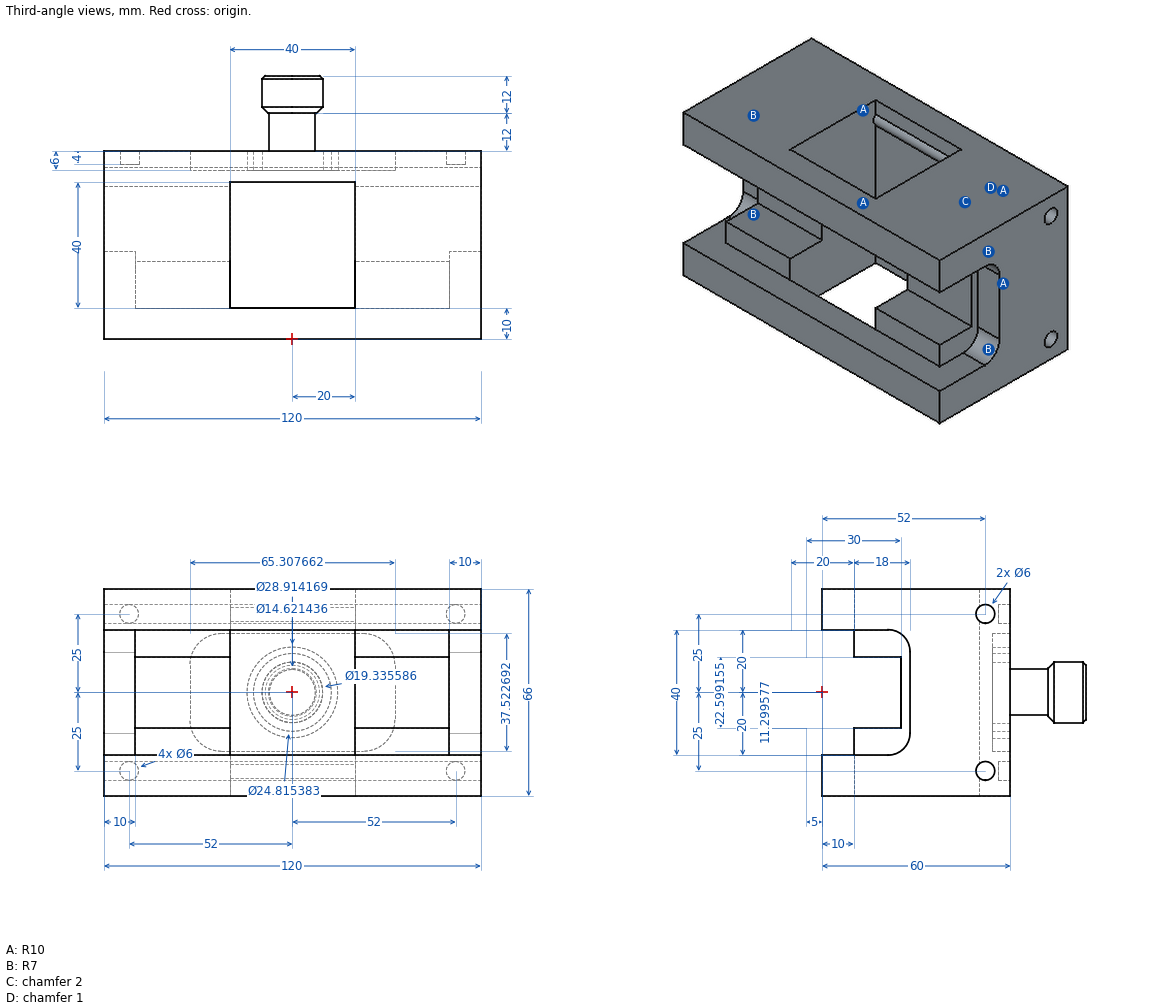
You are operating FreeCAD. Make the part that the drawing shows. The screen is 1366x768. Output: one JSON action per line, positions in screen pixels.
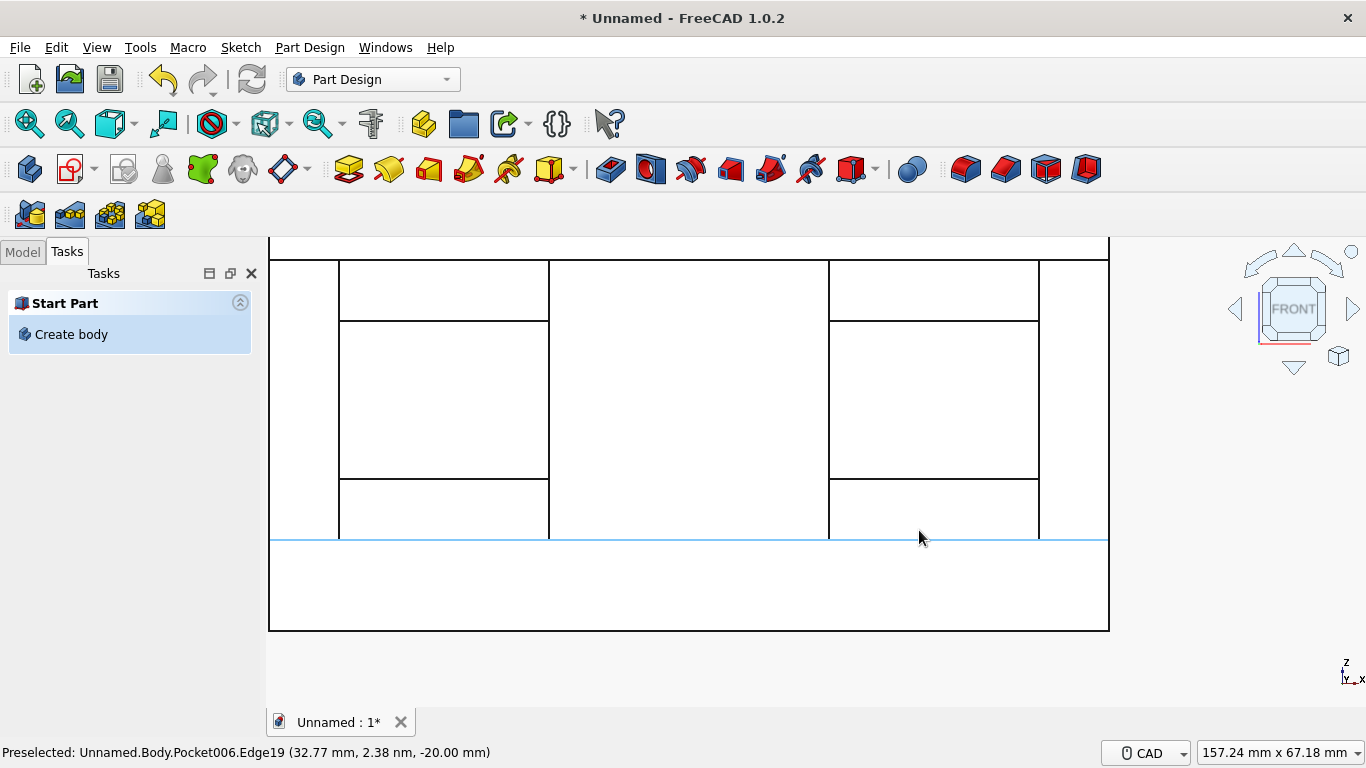
{"action": "left_click", "coordinate": [30, 124]}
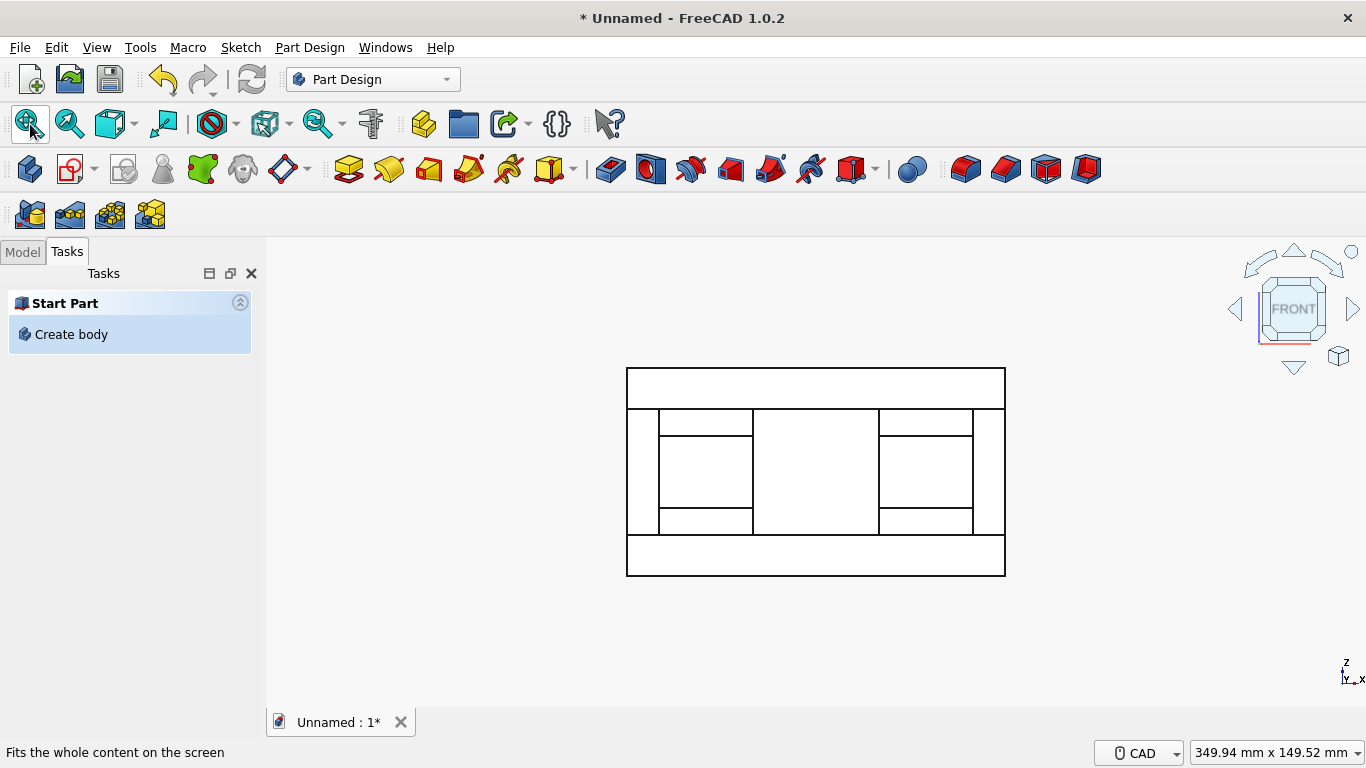
{"action": "key", "text": "3"}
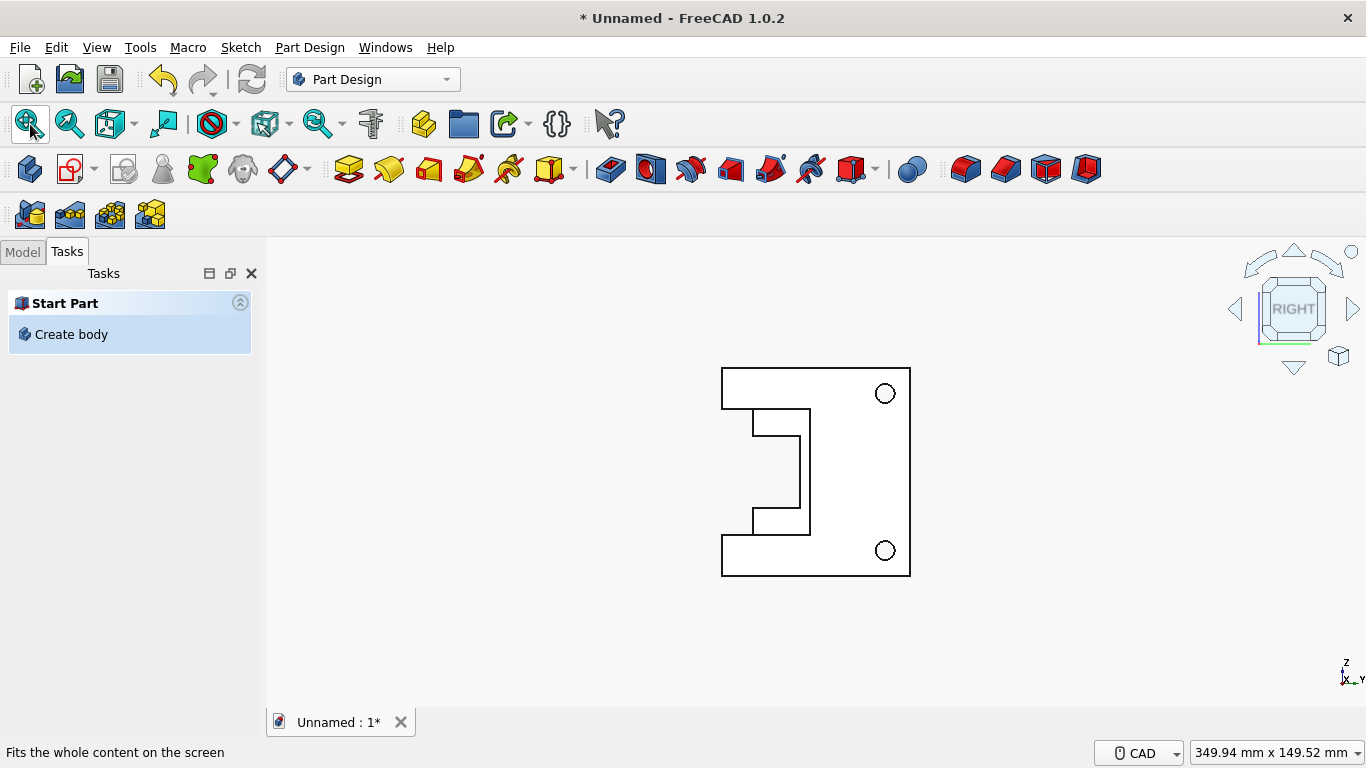
{"action": "left_click", "coordinate": [30, 124]}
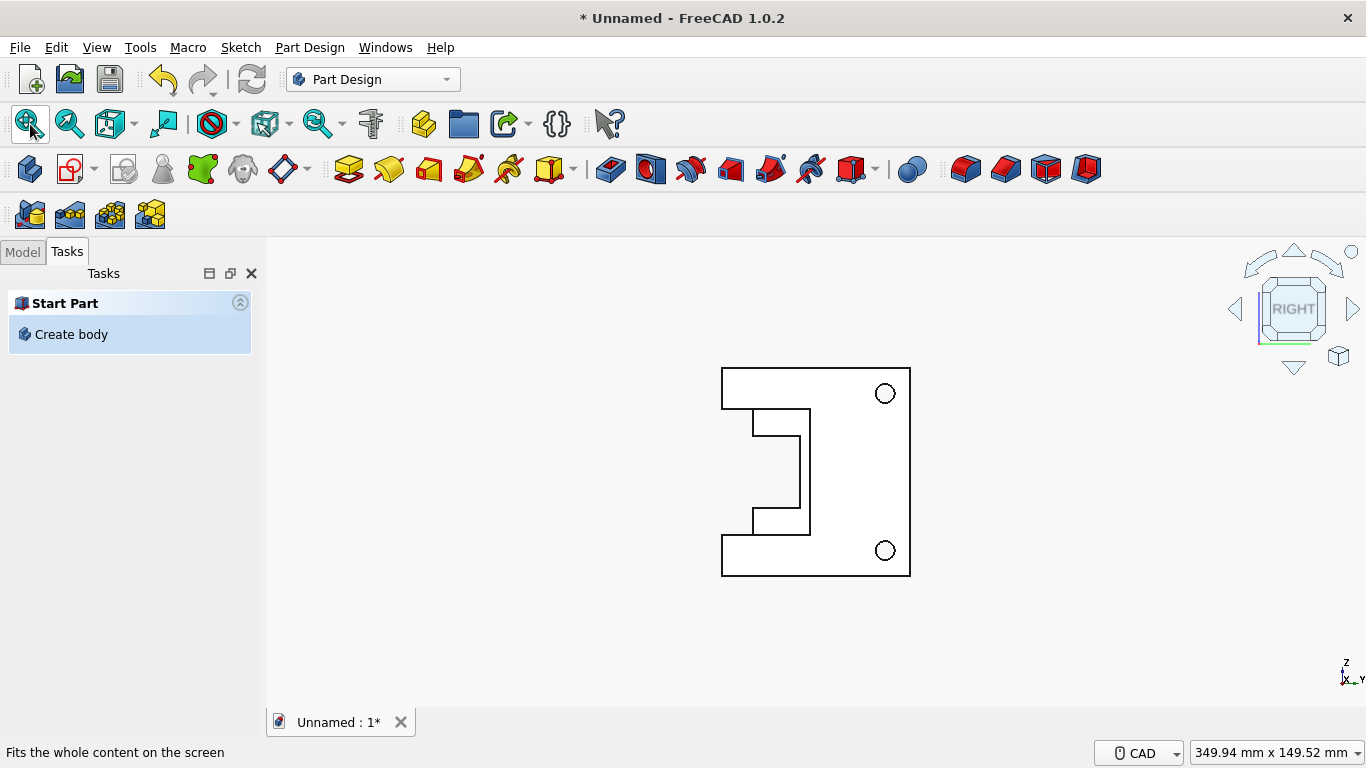
{"action": "scroll", "coordinate": [901, 530], "scroll_direction": "up", "scroll_amount": 4}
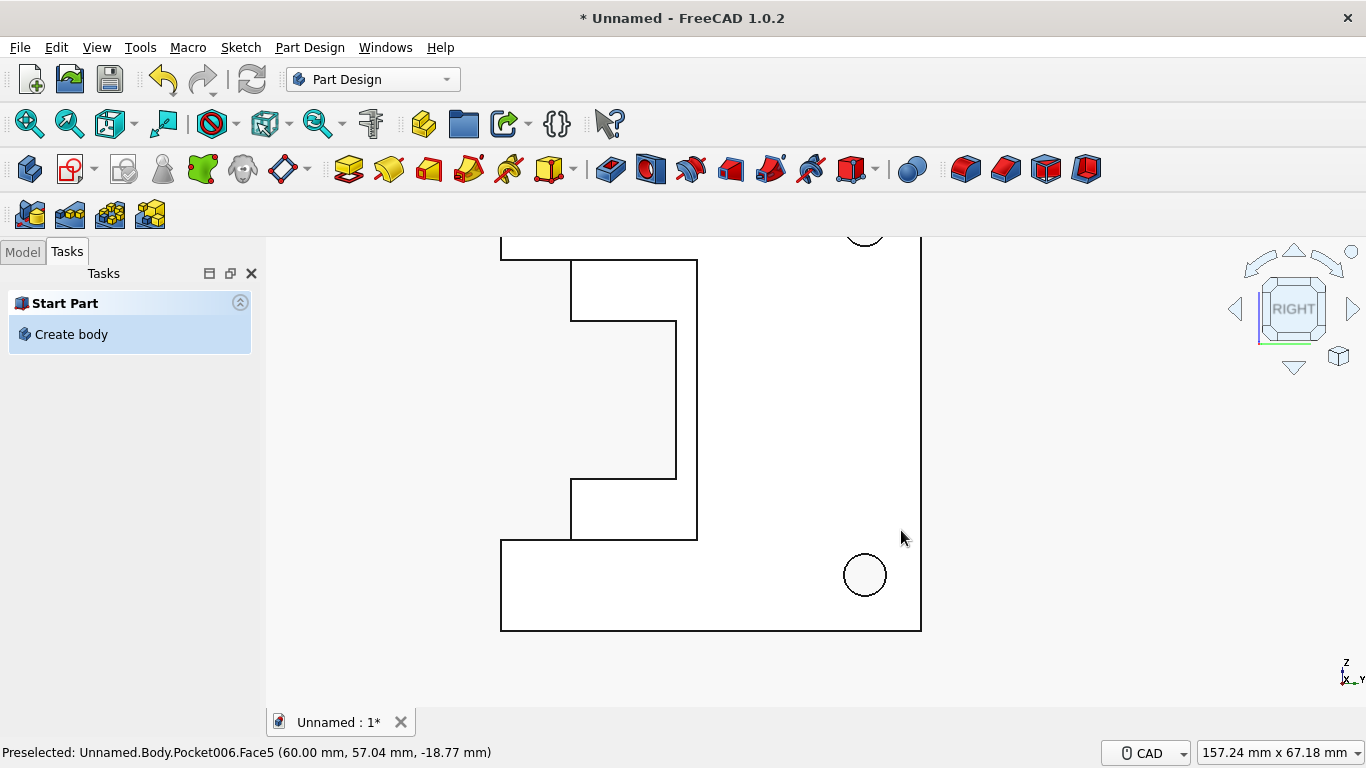
{"action": "left_click", "coordinate": [30, 124]}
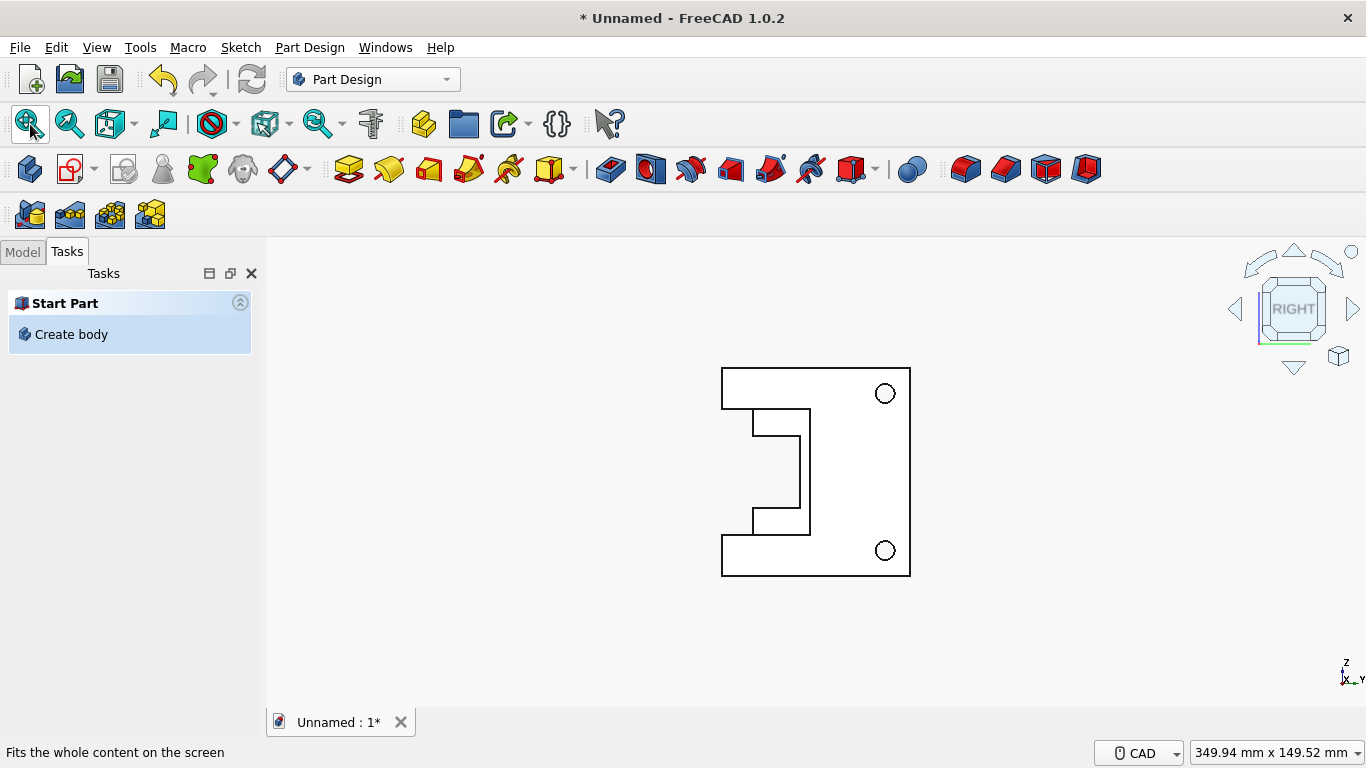
{"action": "key", "text": "5"}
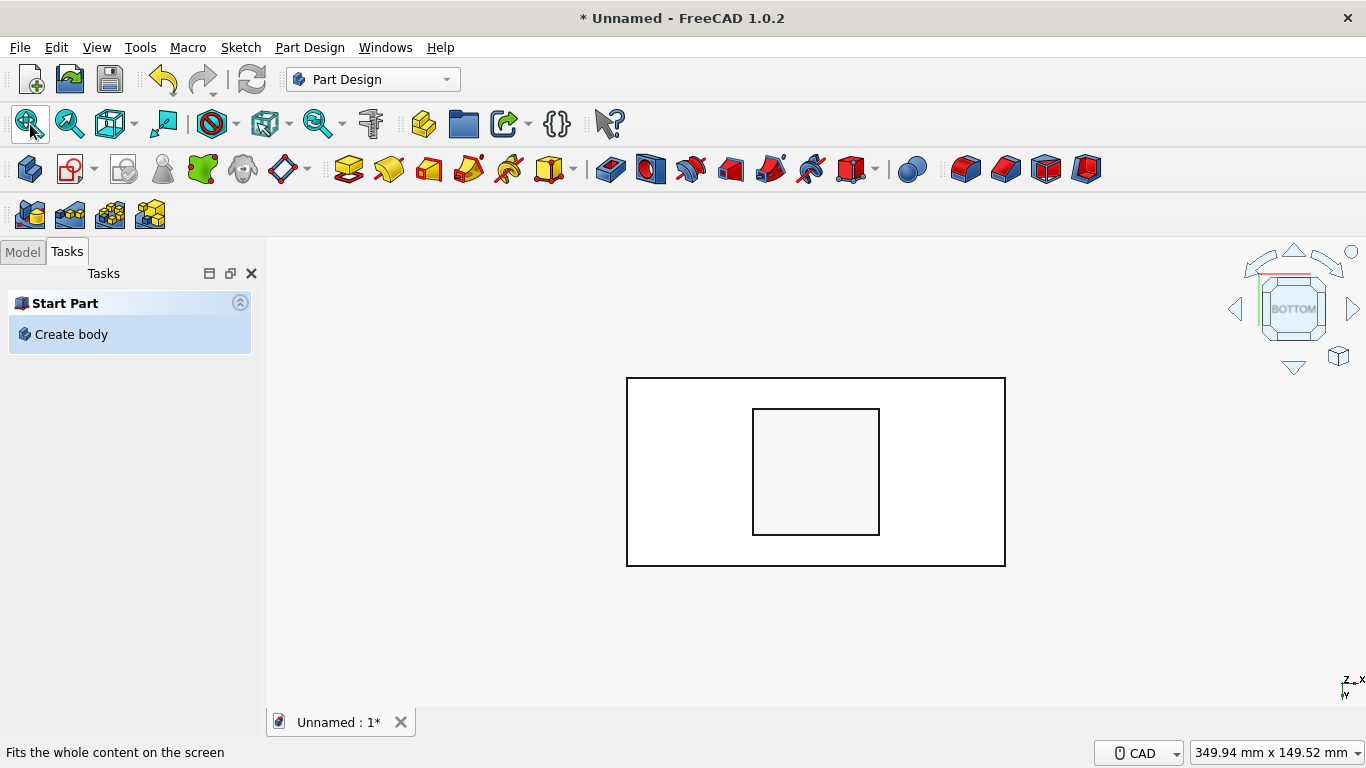
{"action": "left_click", "coordinate": [30, 124]}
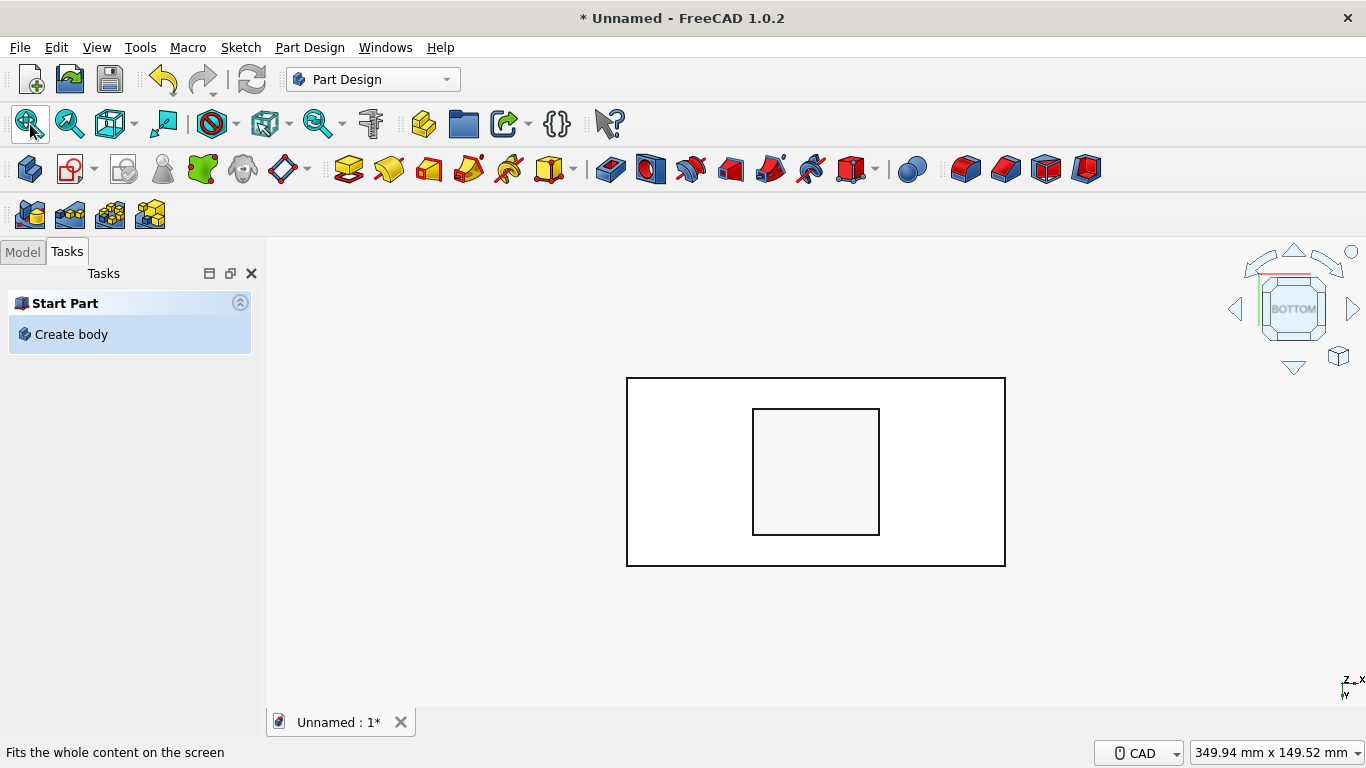
{"action": "scroll", "coordinate": [919, 556], "scroll_direction": "up", "scroll_amount": 4}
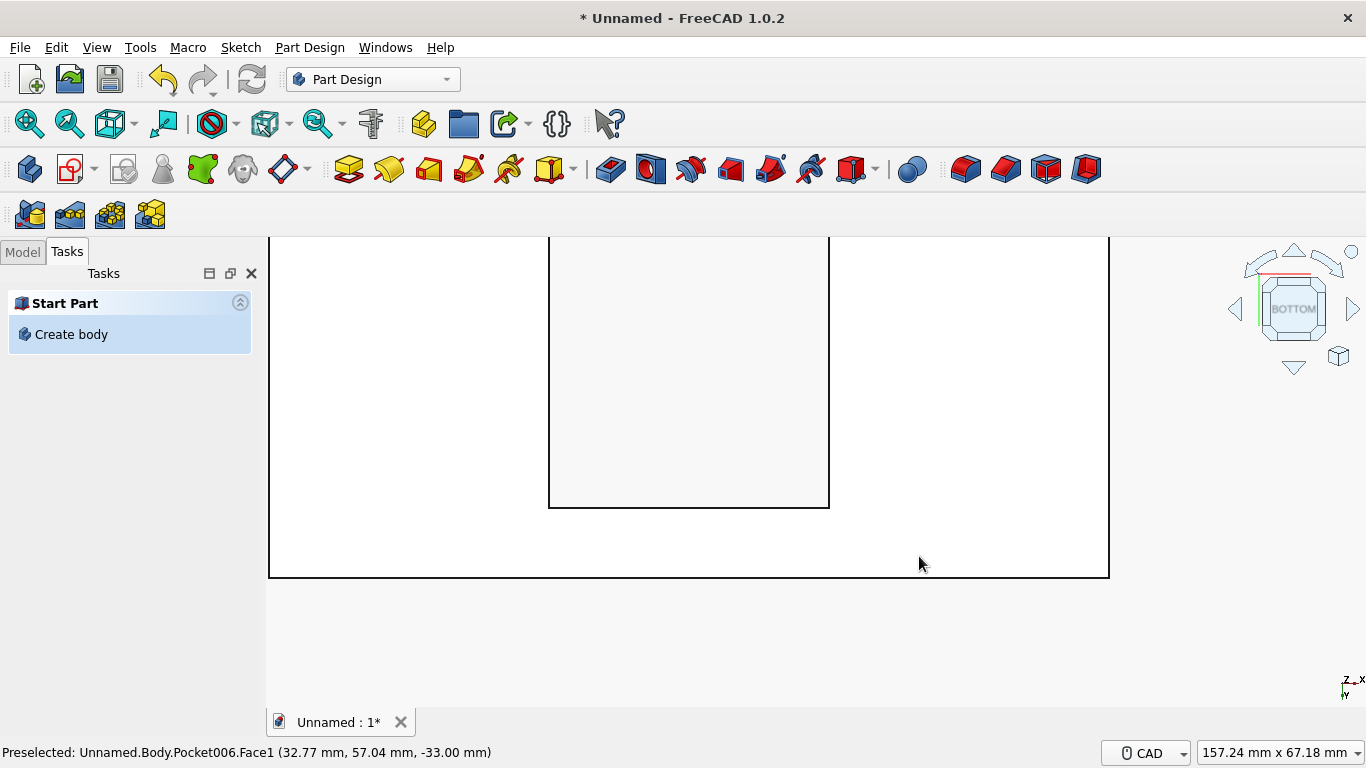
{"action": "left_click", "coordinate": [30, 124]}